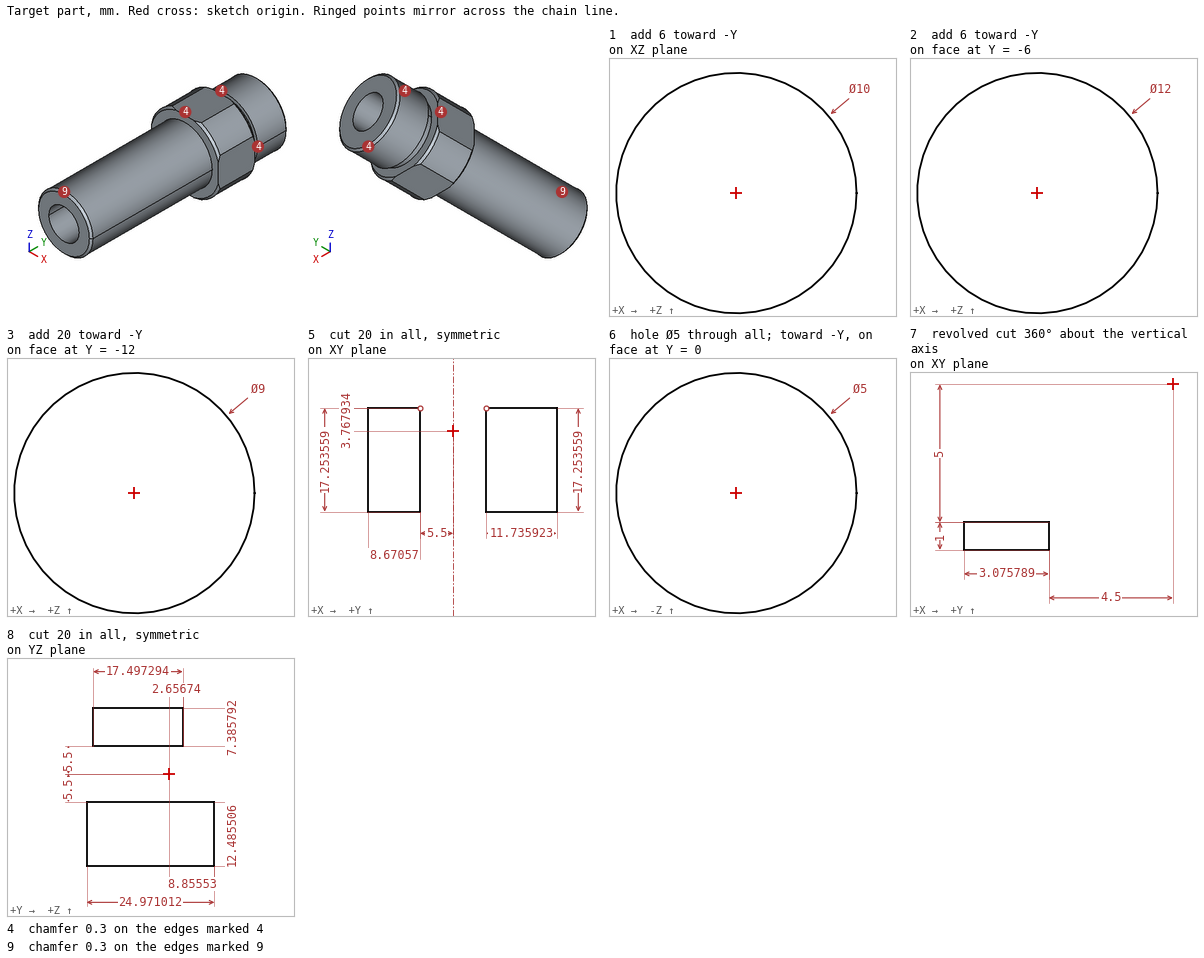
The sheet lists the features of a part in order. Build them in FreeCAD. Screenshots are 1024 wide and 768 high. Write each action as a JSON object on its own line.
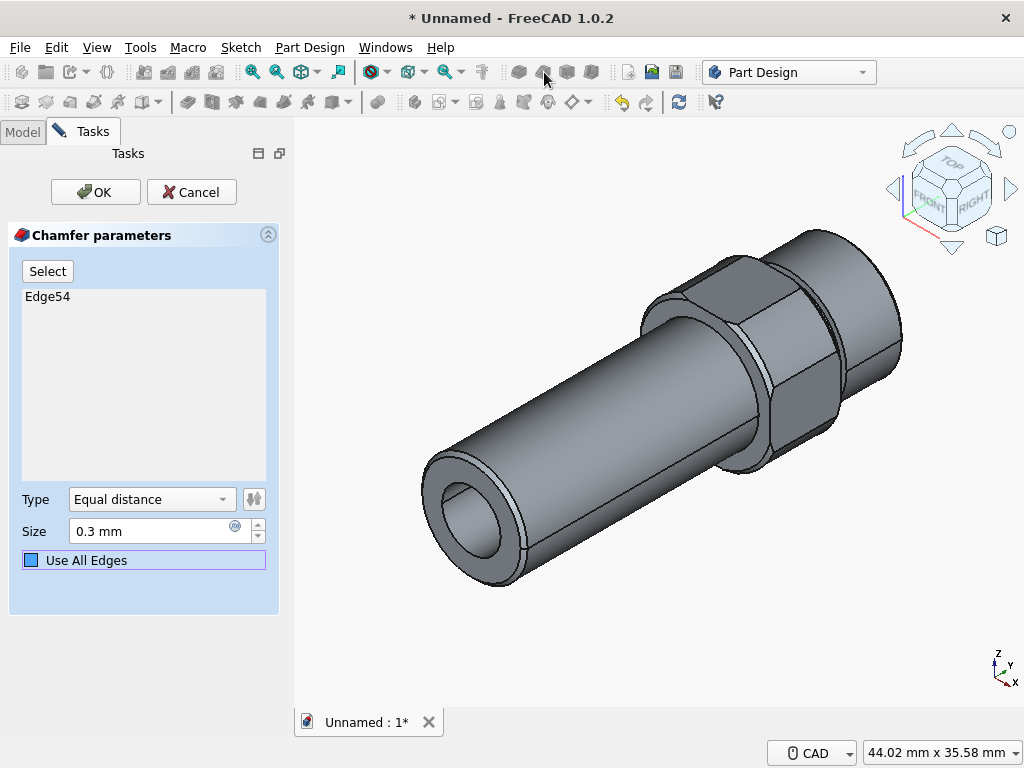
{"action": "left_click", "coordinate": [96, 192]}